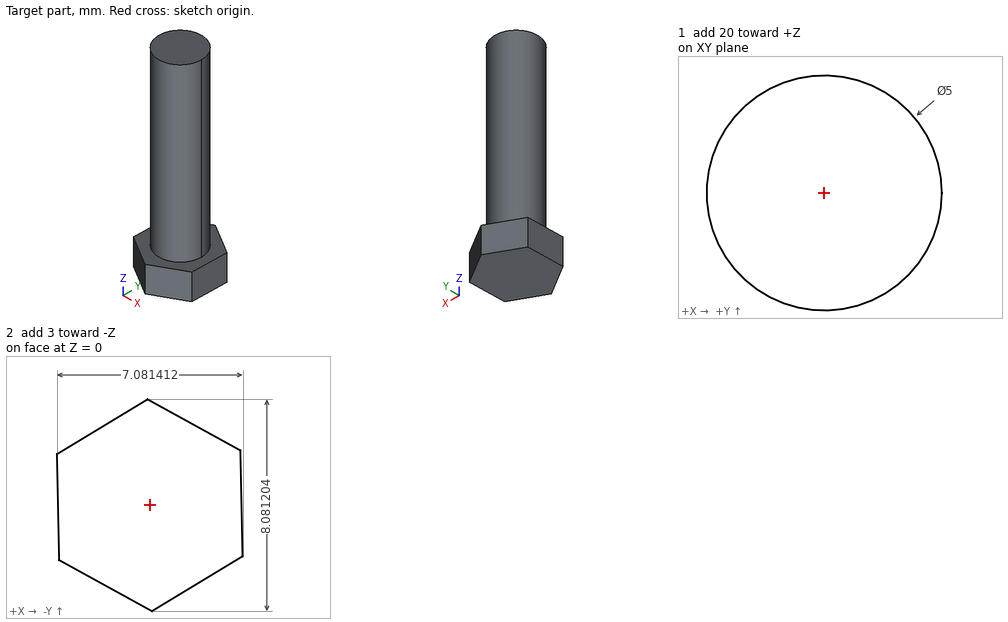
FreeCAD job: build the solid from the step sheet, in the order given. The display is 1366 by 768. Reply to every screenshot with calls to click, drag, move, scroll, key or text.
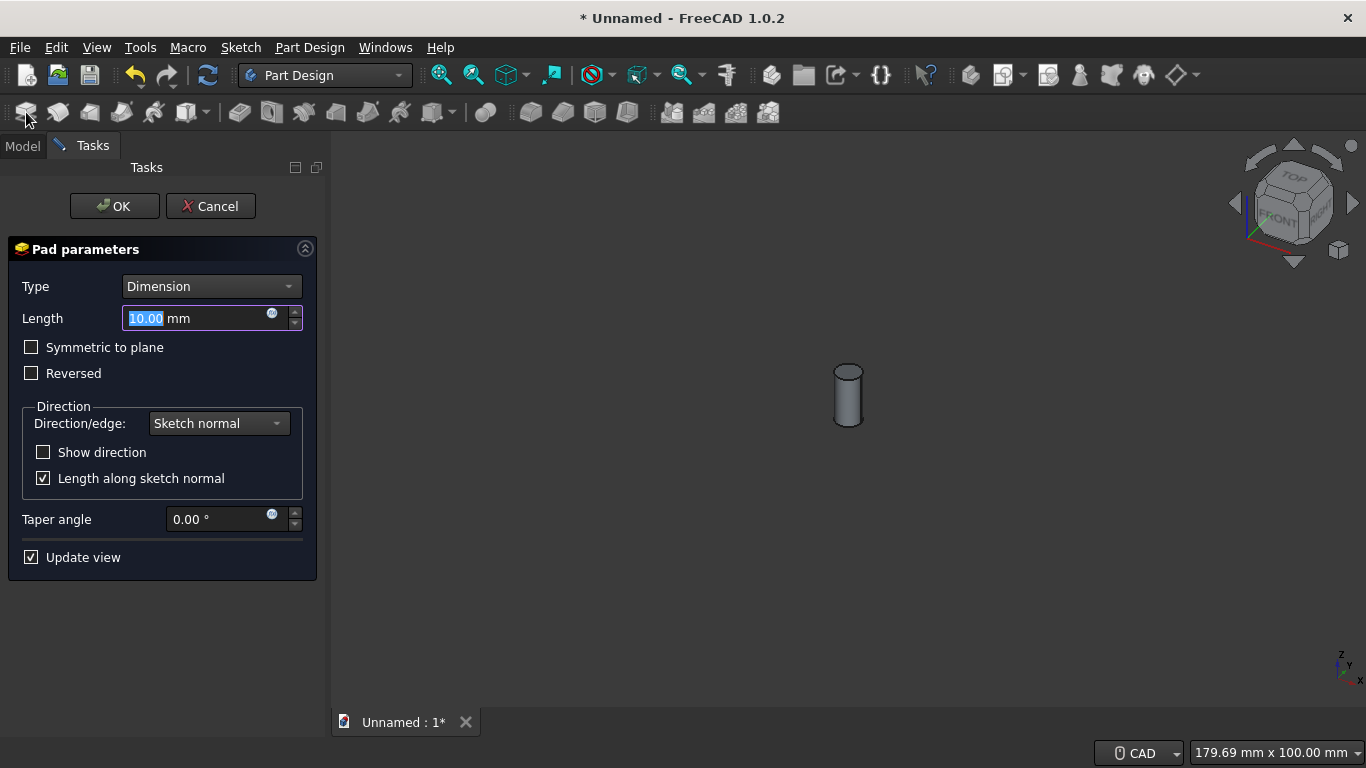
text(20)
key(Tab)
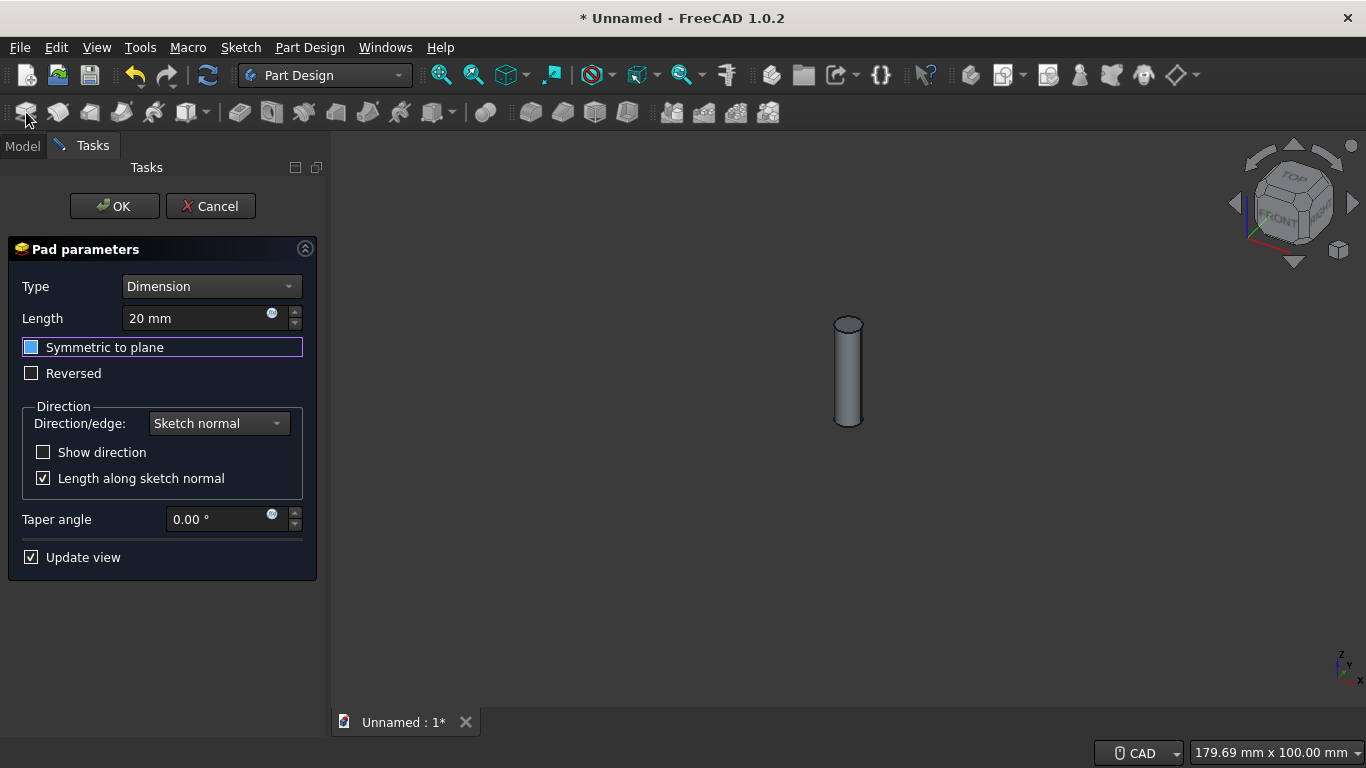
click(115, 206)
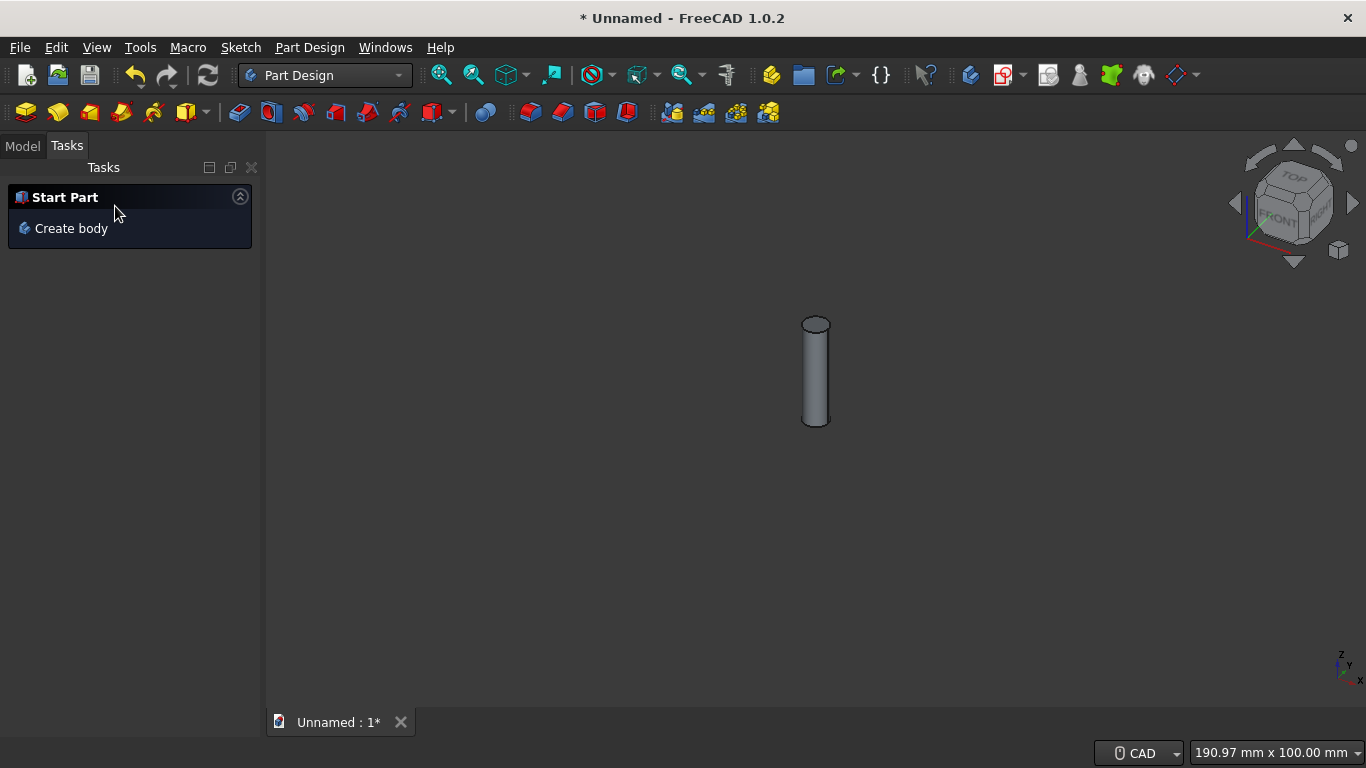
key(v)
key(f)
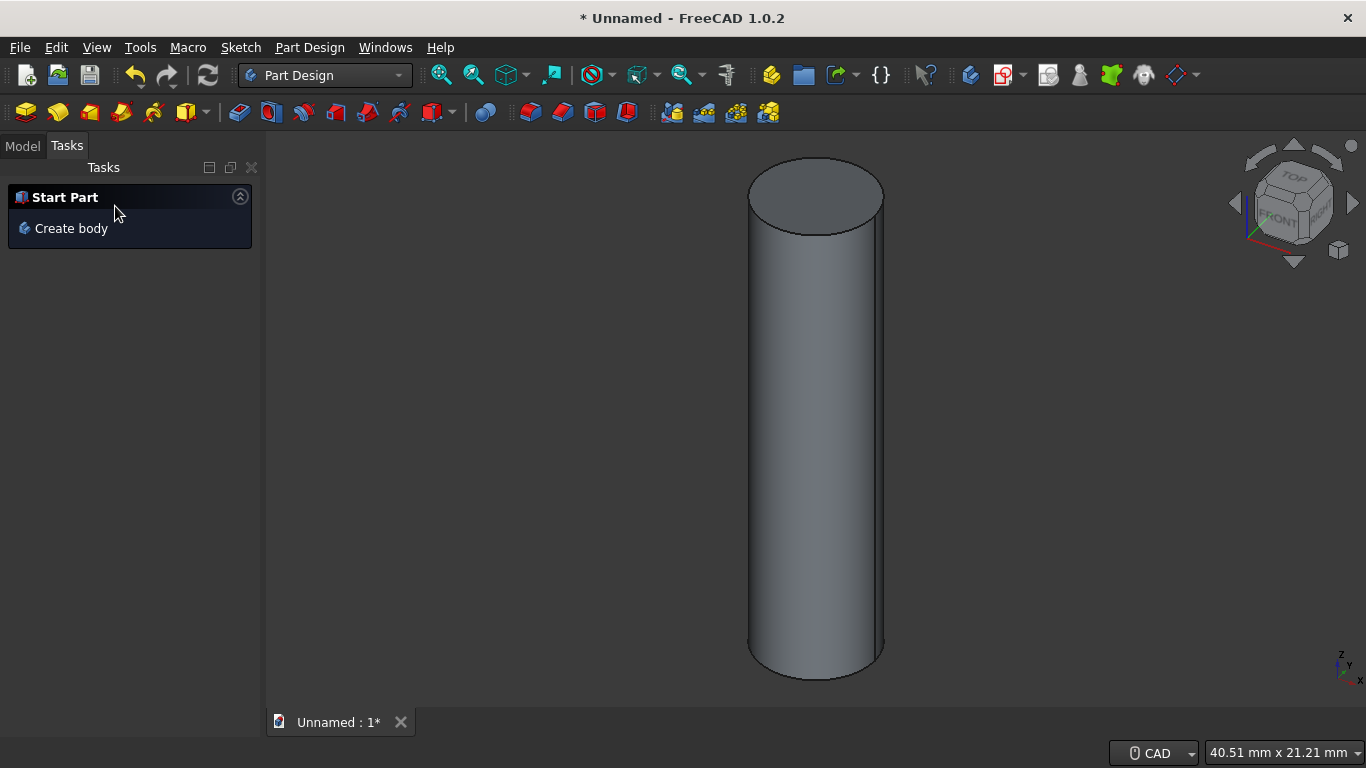
key(5)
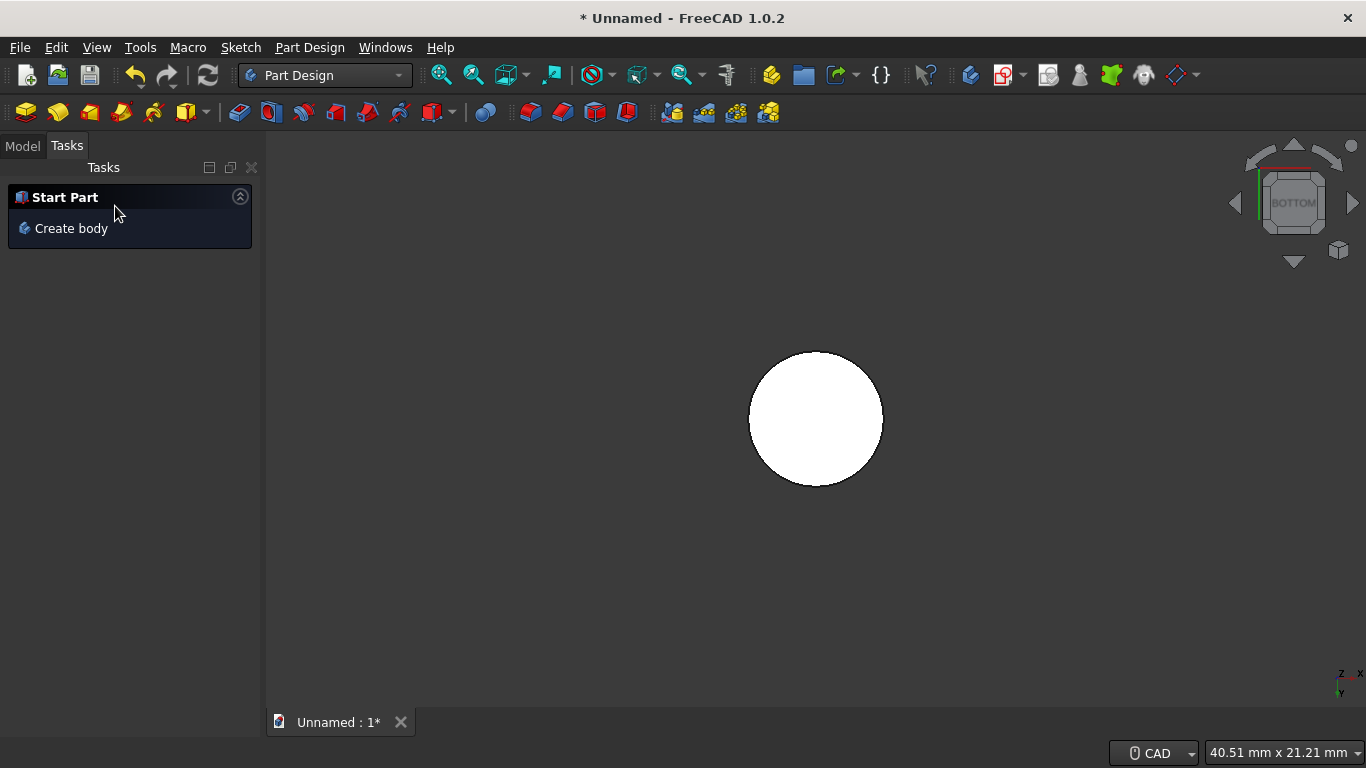
click(442, 76)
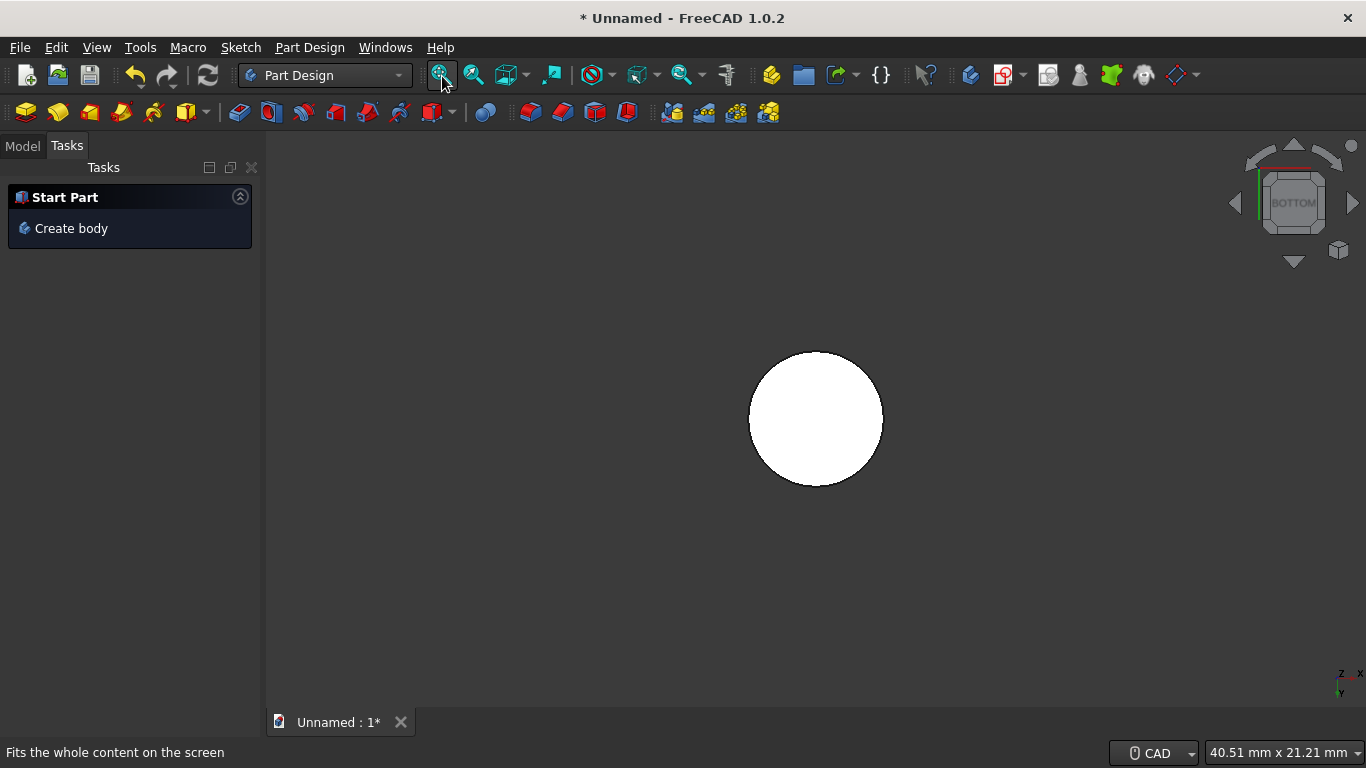
click(816, 418)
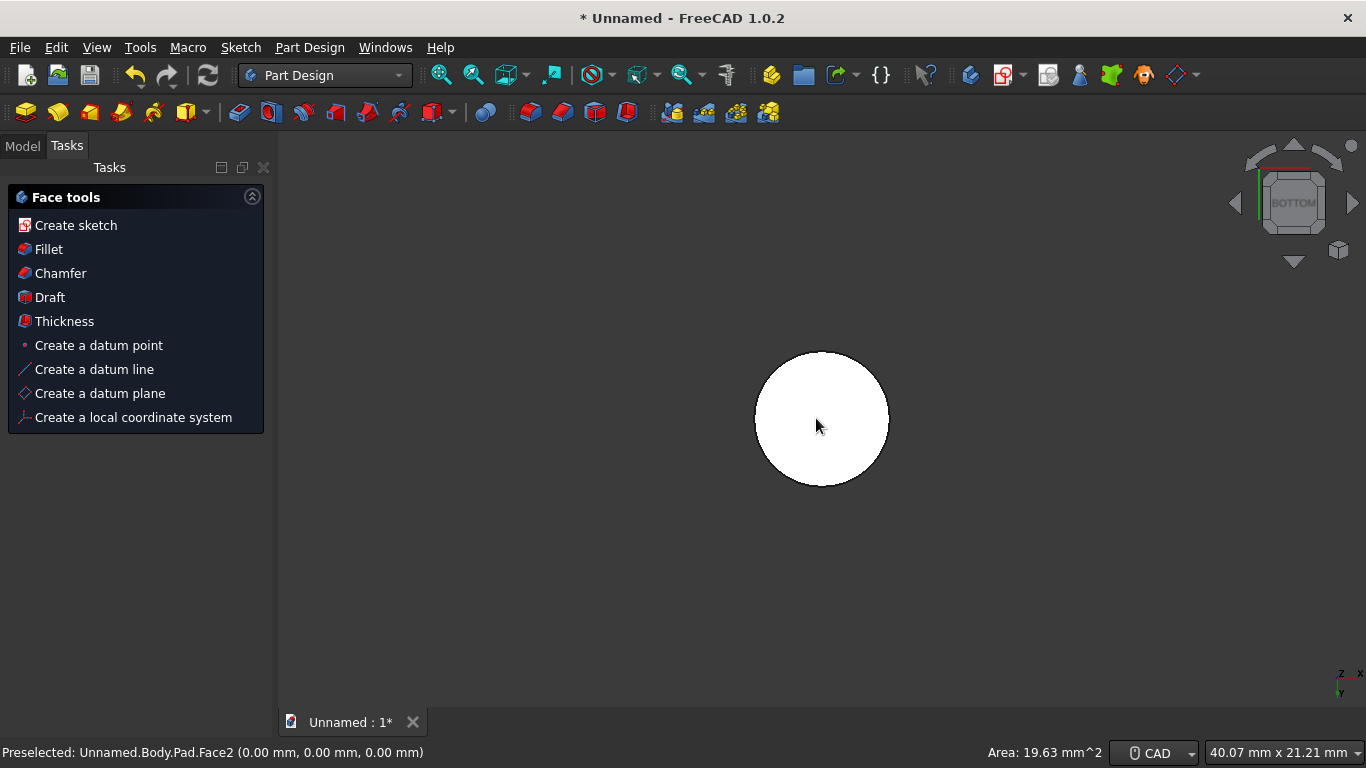
click(1004, 76)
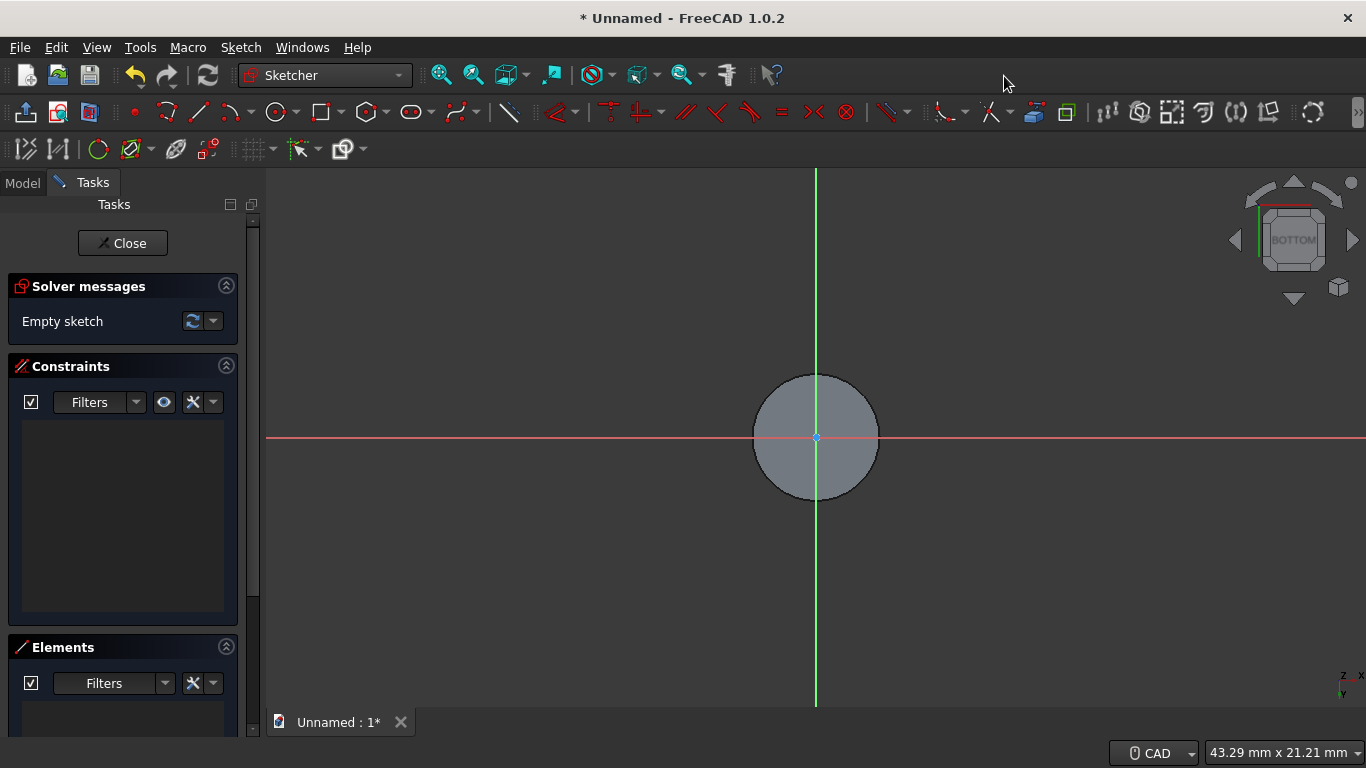
scroll(899, 438, up, 3)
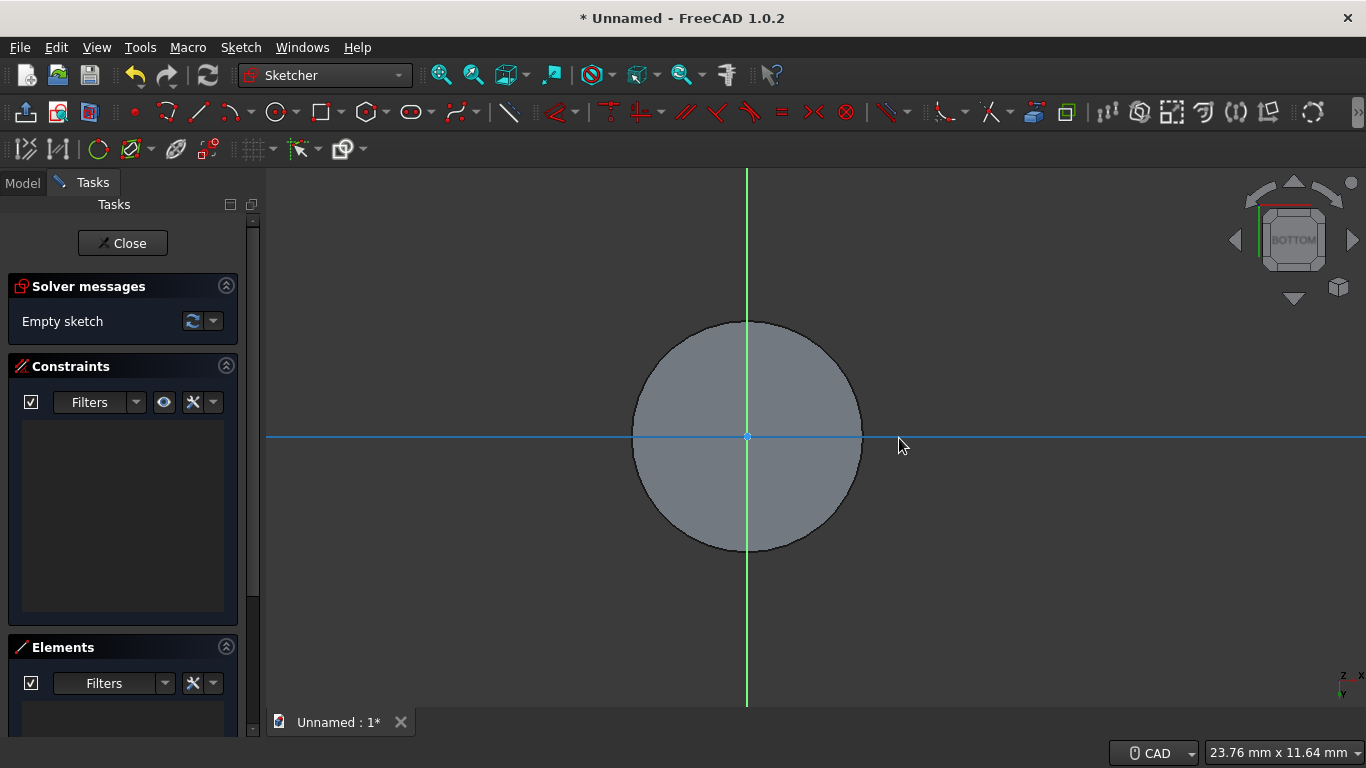
click(366, 112)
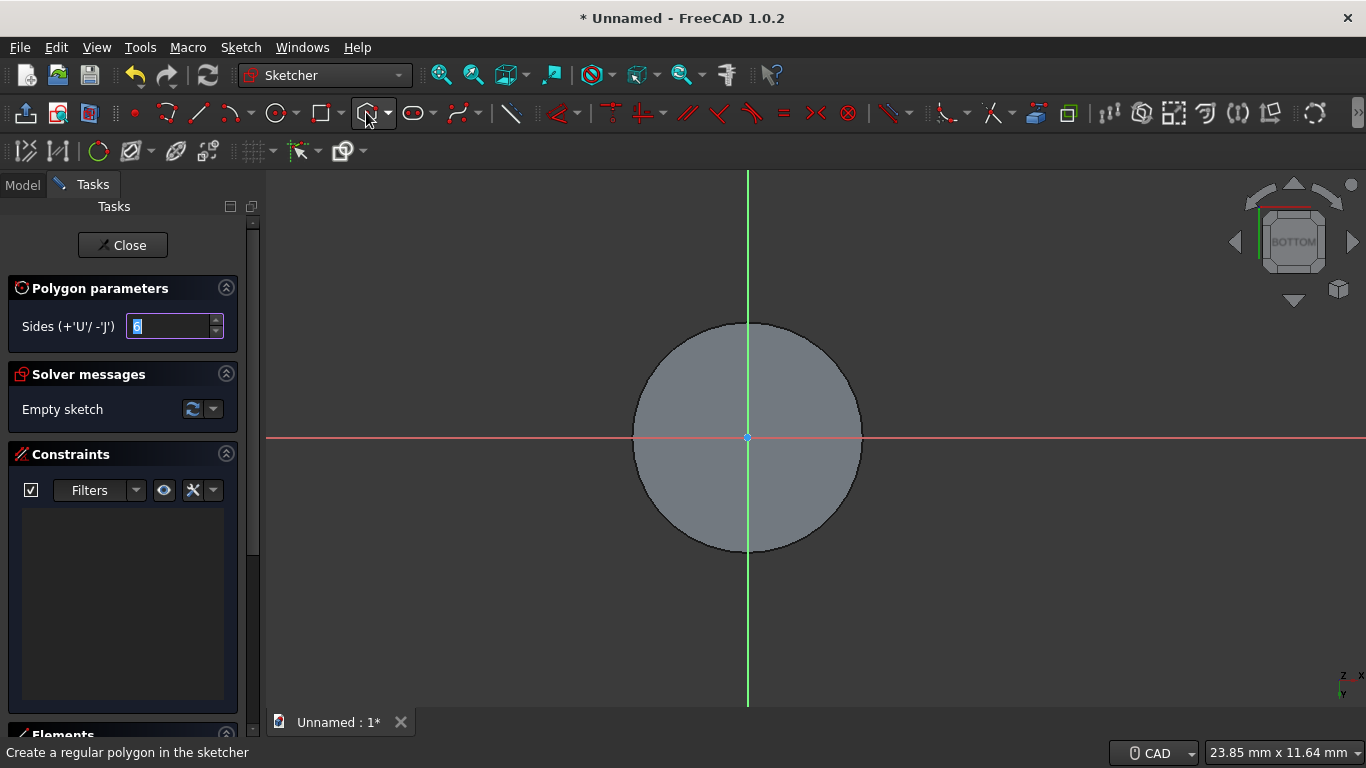
click(748, 438)